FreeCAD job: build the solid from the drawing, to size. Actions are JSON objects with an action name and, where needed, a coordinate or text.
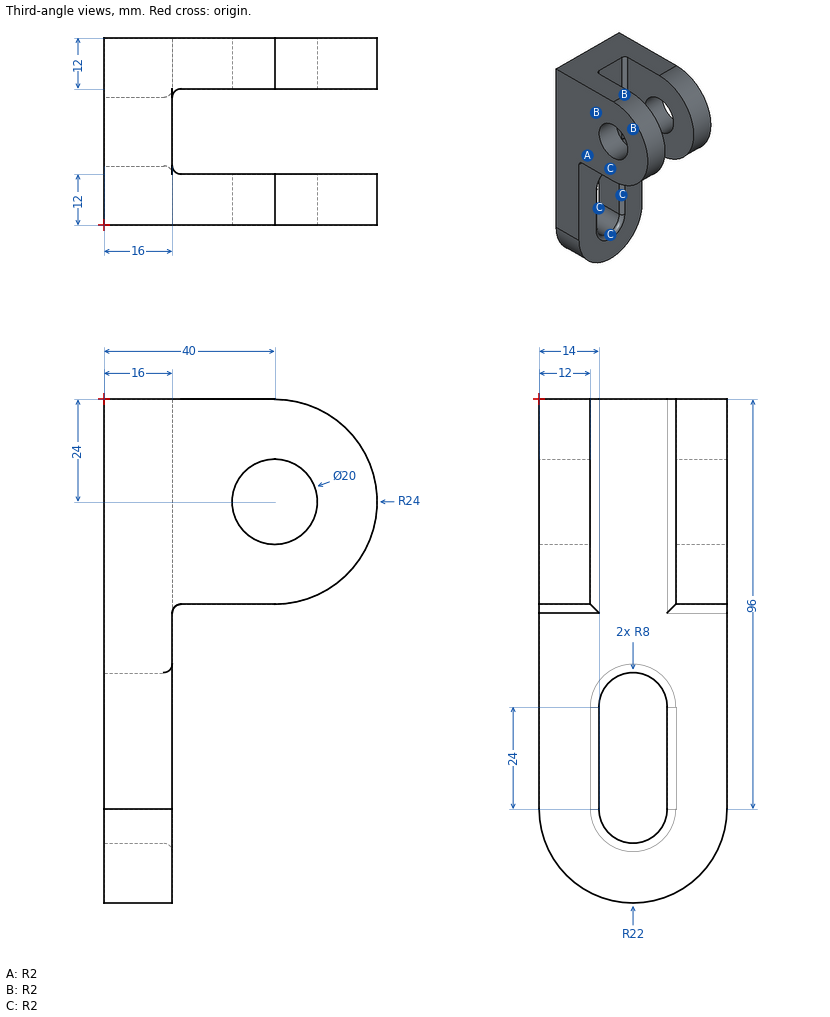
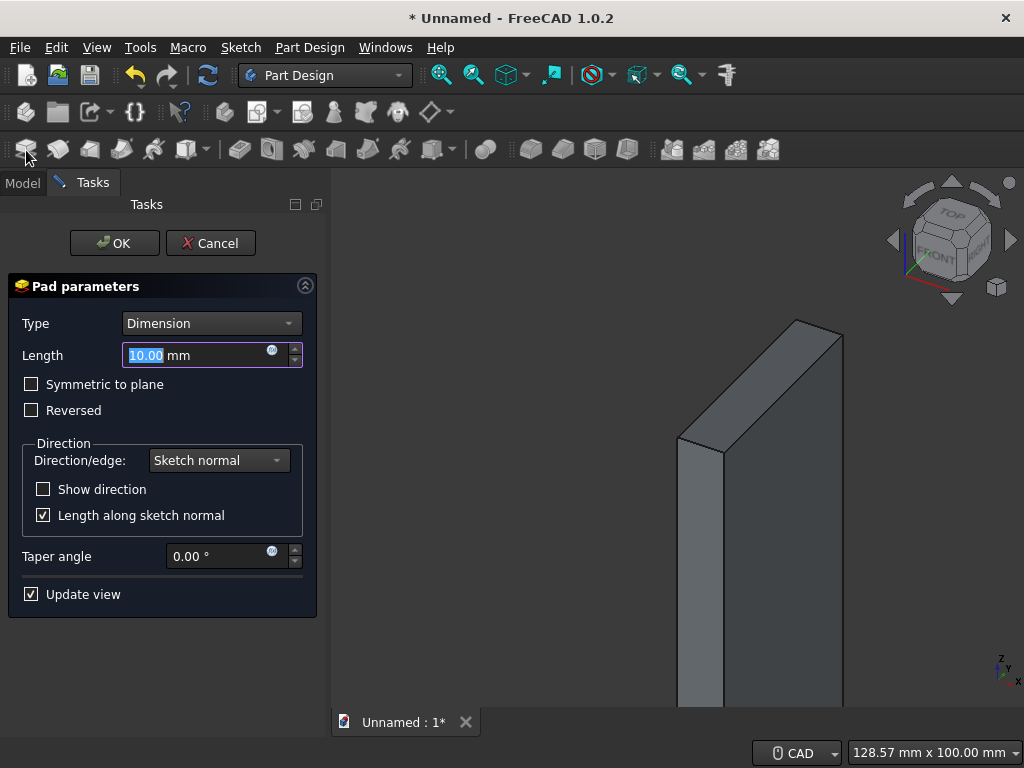
{"action": "type", "text": "16"}
{"action": "key", "text": "Tab"}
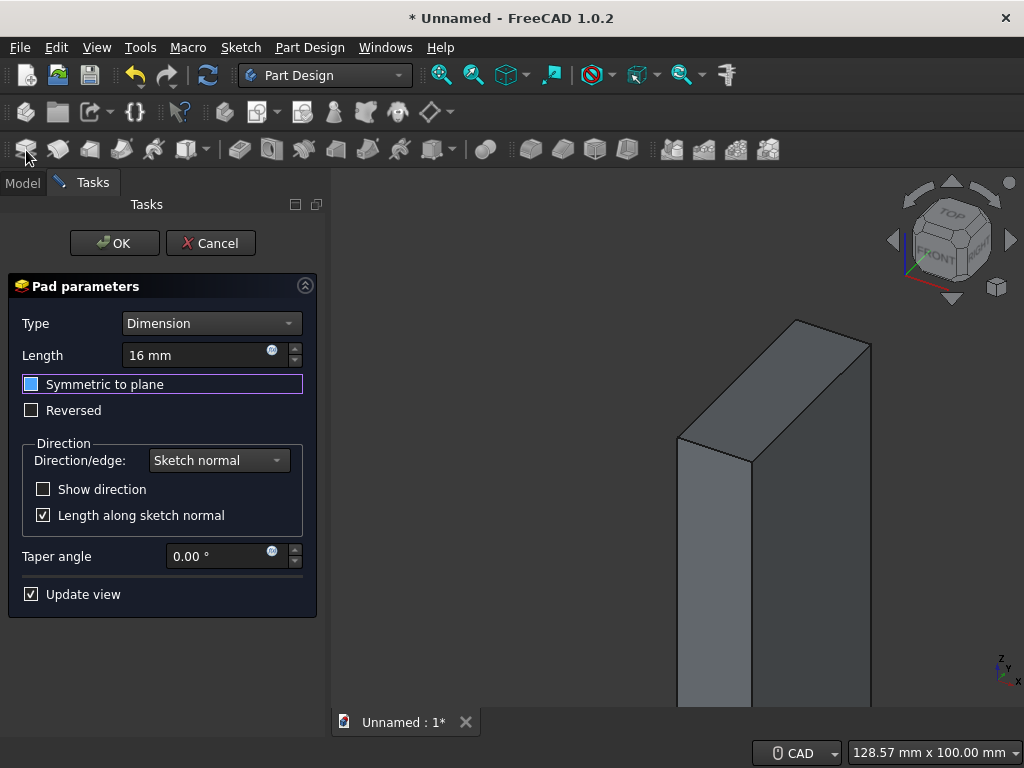
{"action": "left_click", "coordinate": [115, 243]}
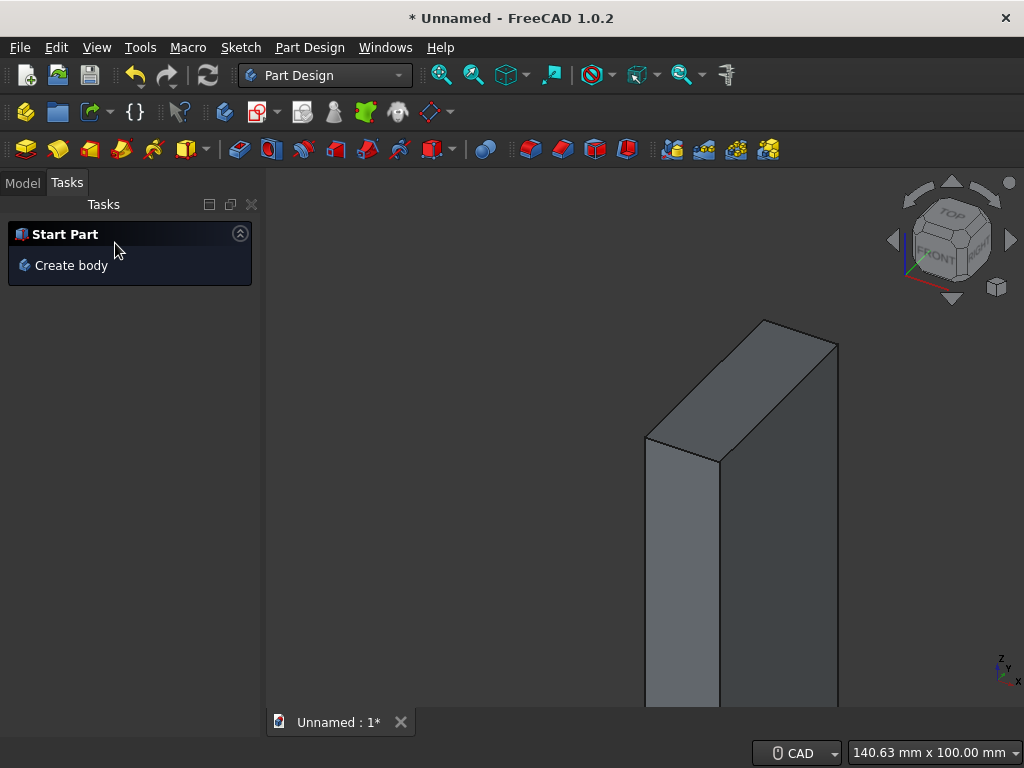
{"action": "left_click", "coordinate": [442, 76]}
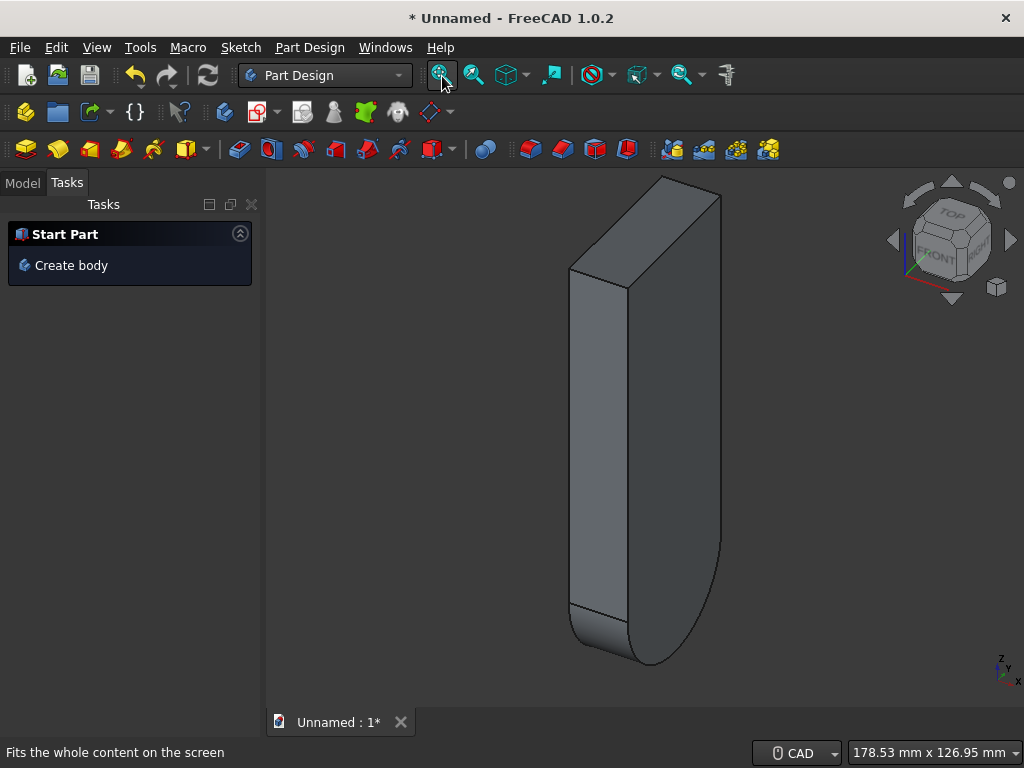
{"action": "left_click", "coordinate": [674, 563]}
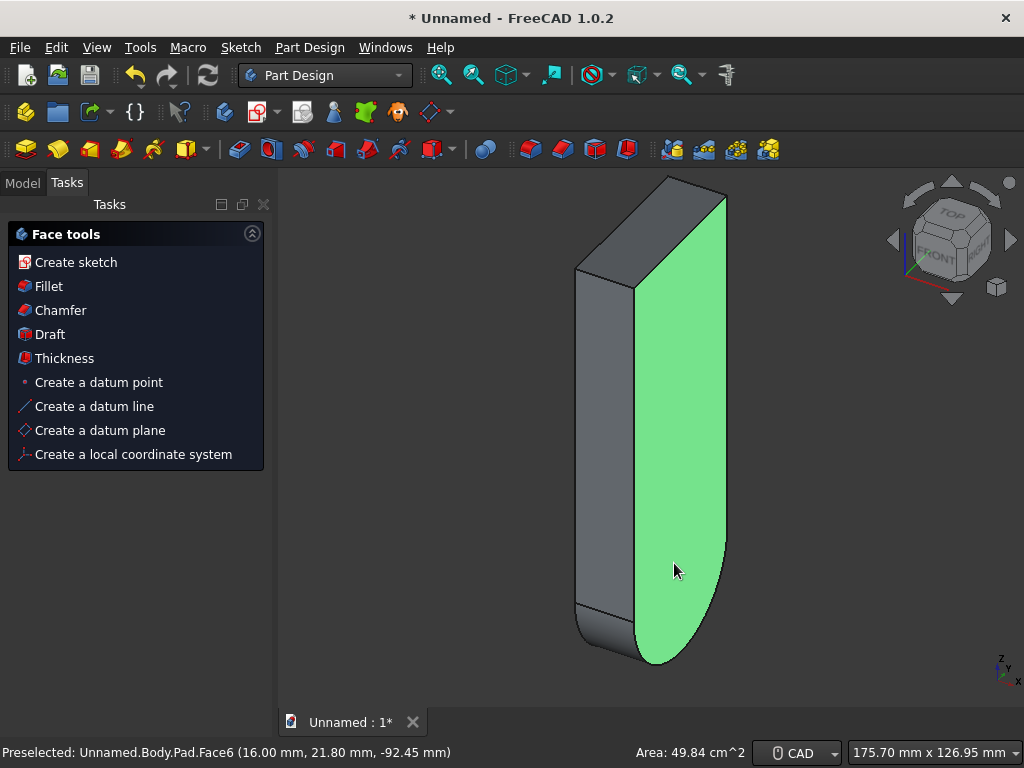
{"action": "left_click", "coordinate": [258, 112]}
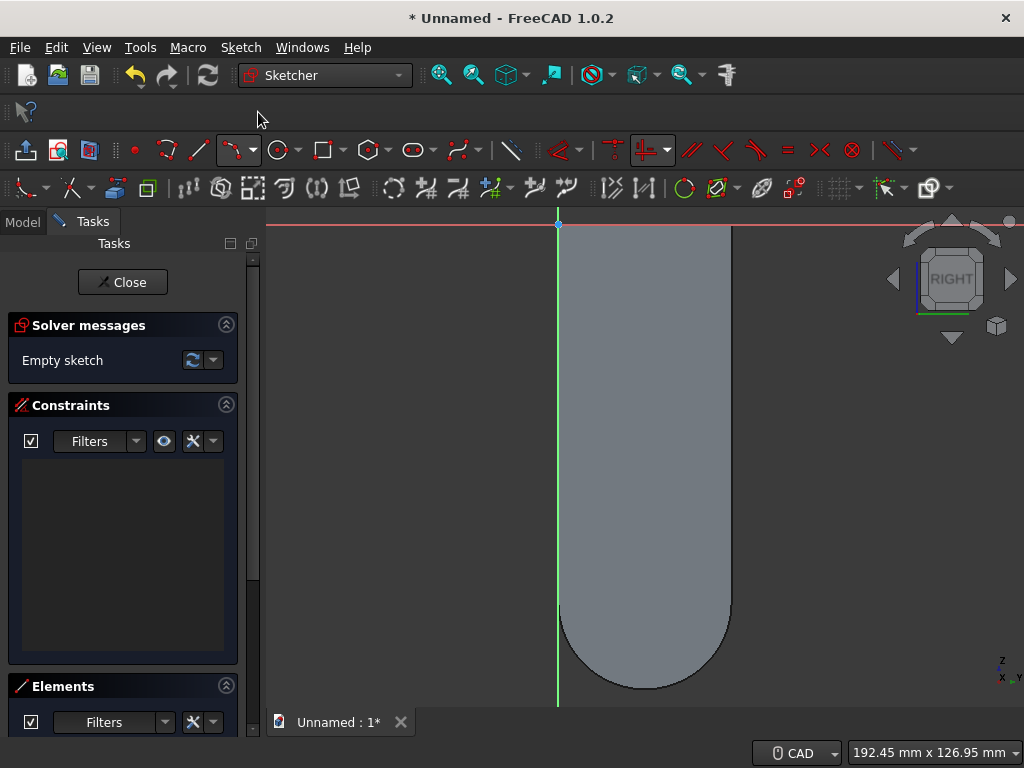
{"action": "scroll", "coordinate": [728, 675], "scroll_direction": "up", "scroll_amount": 3}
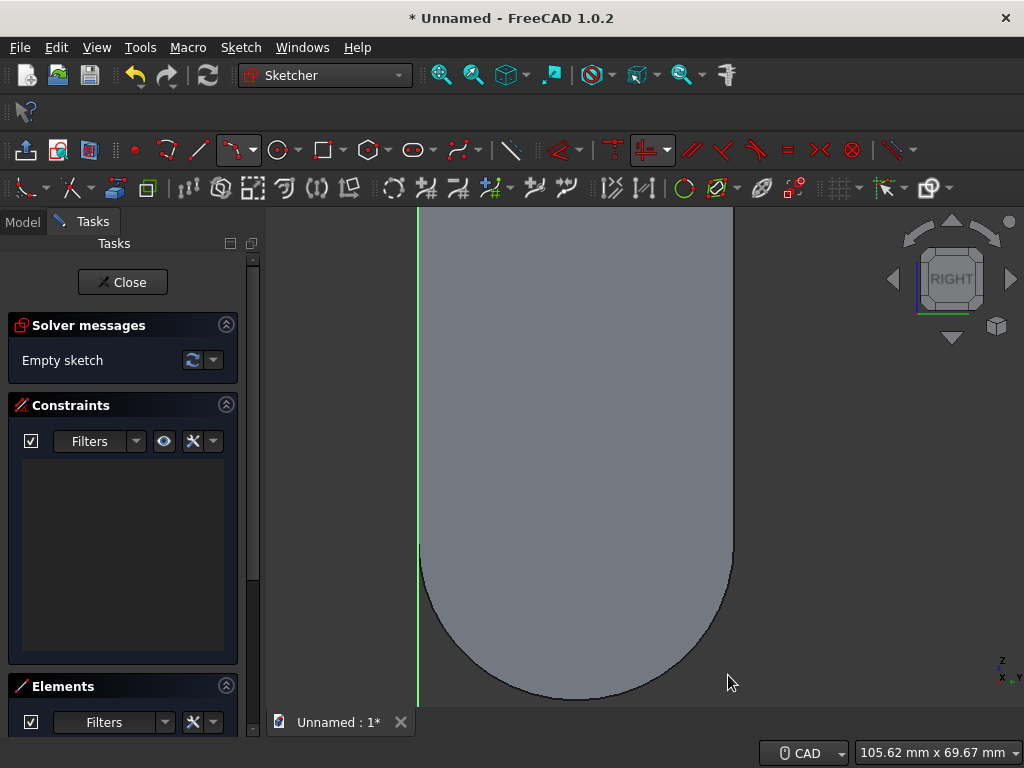
{"action": "left_click", "coordinate": [414, 150]}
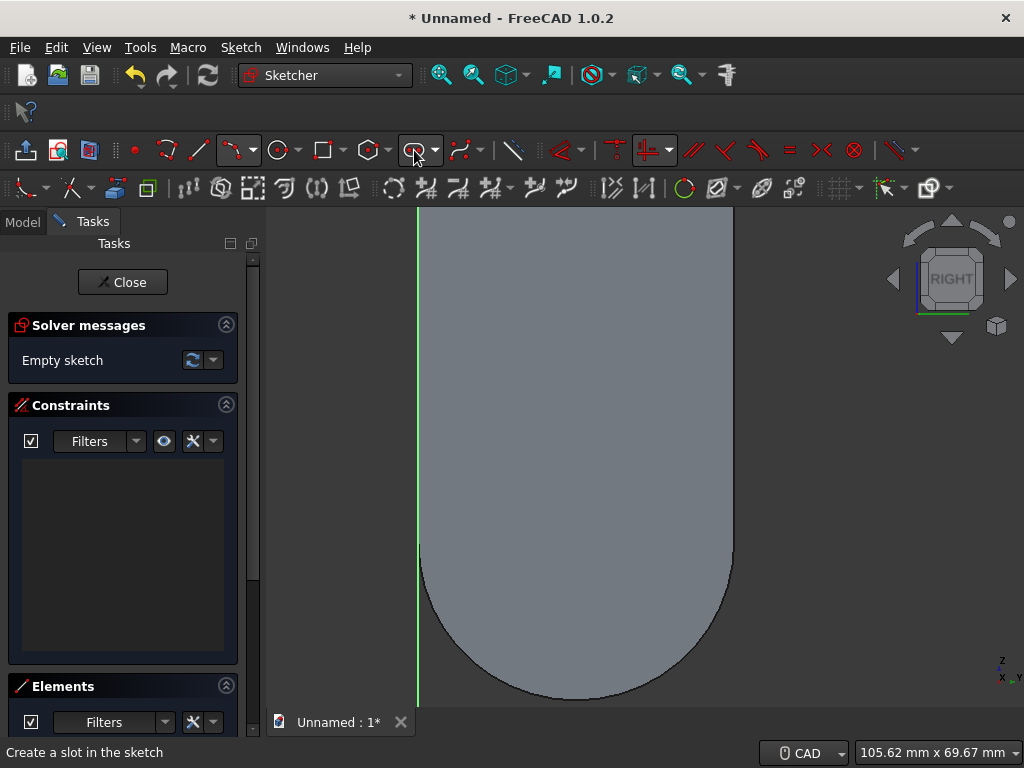
{"action": "left_click", "coordinate": [576, 543]}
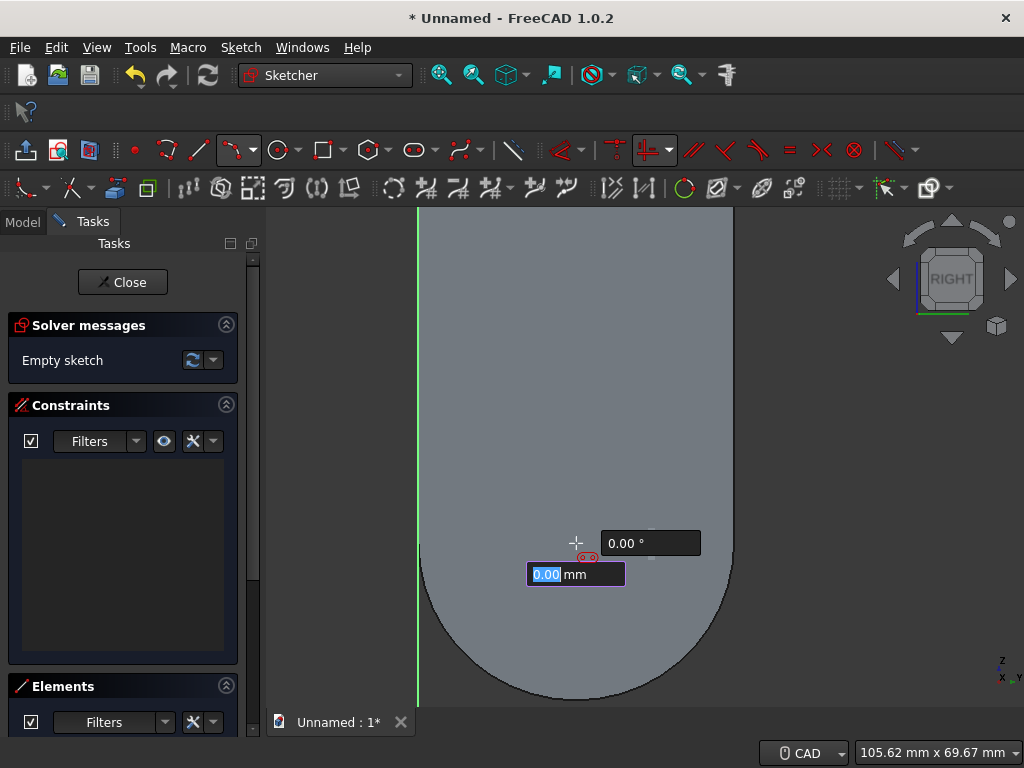
{"action": "left_click", "coordinate": [576, 370]}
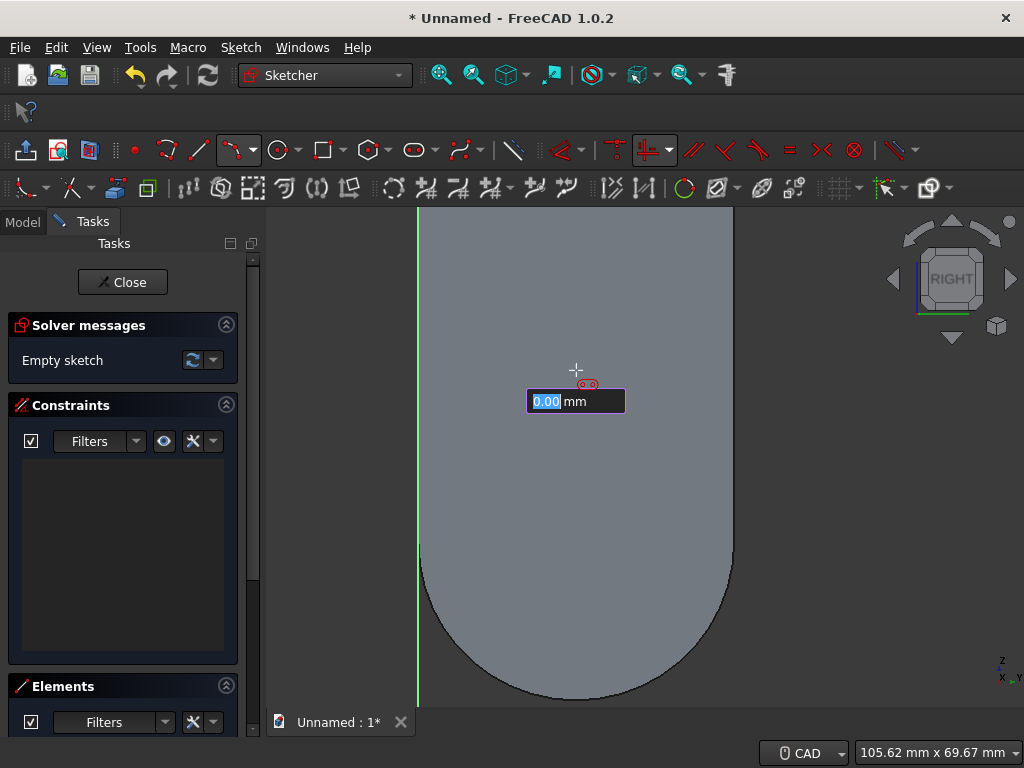
{"action": "left_click", "coordinate": [634, 456]}
{"action": "key", "text": "Escape"}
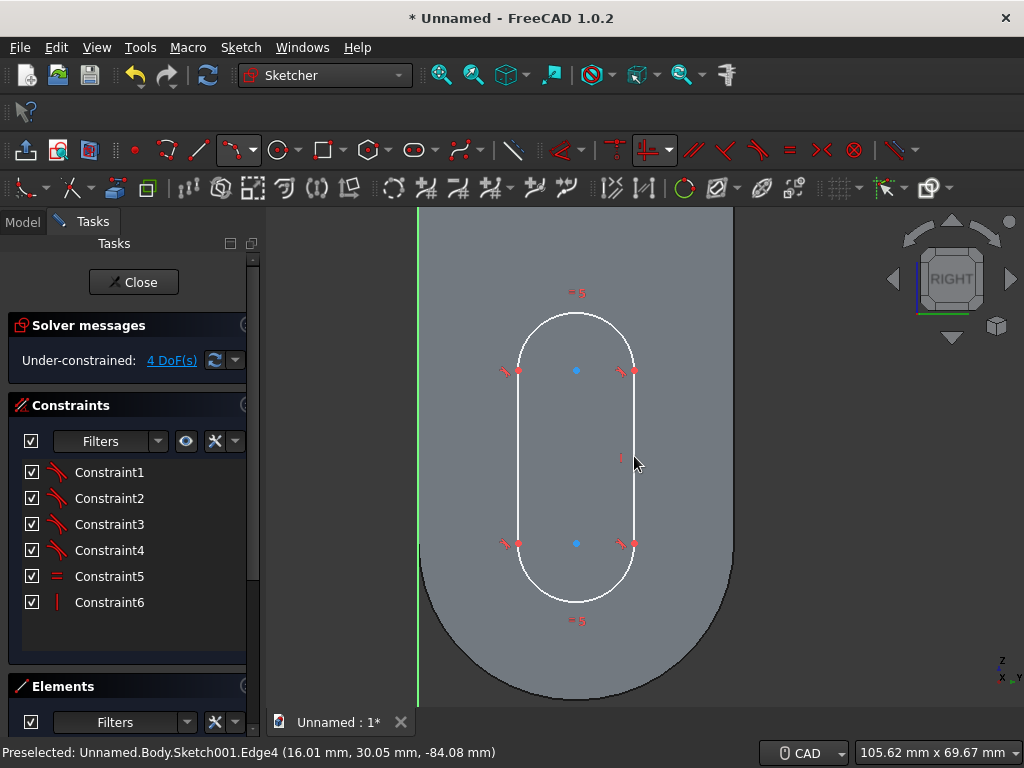
{"action": "left_click", "coordinate": [560, 150]}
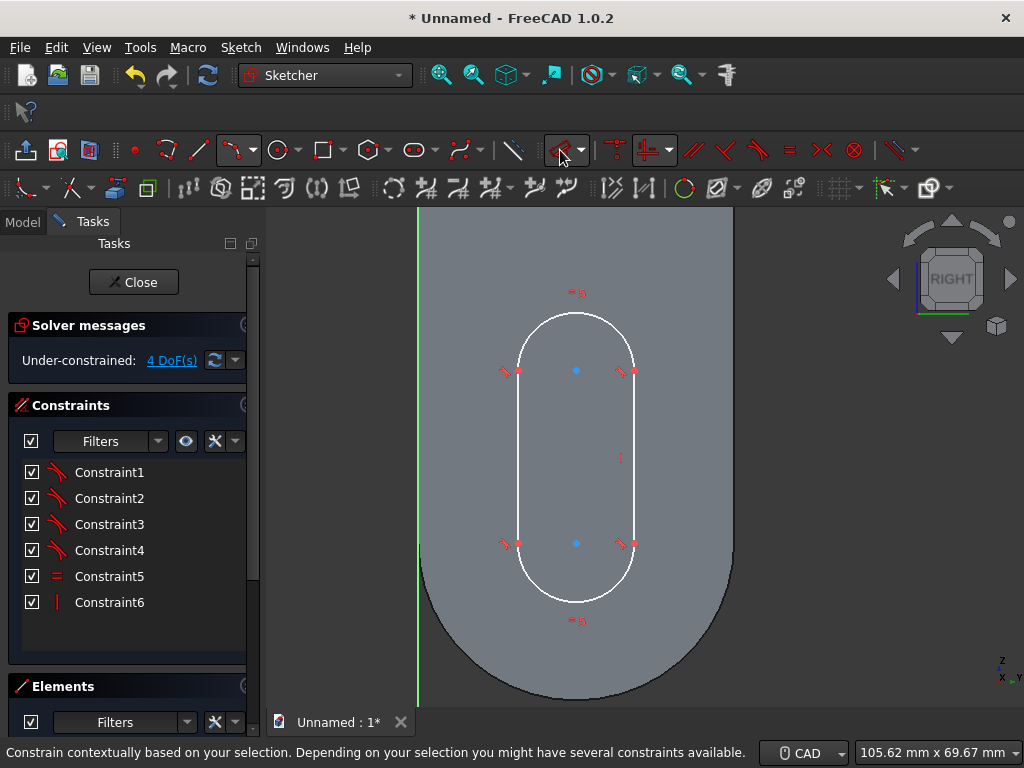
{"action": "left_click", "coordinate": [542, 591]}
{"action": "left_click", "coordinate": [523, 617]}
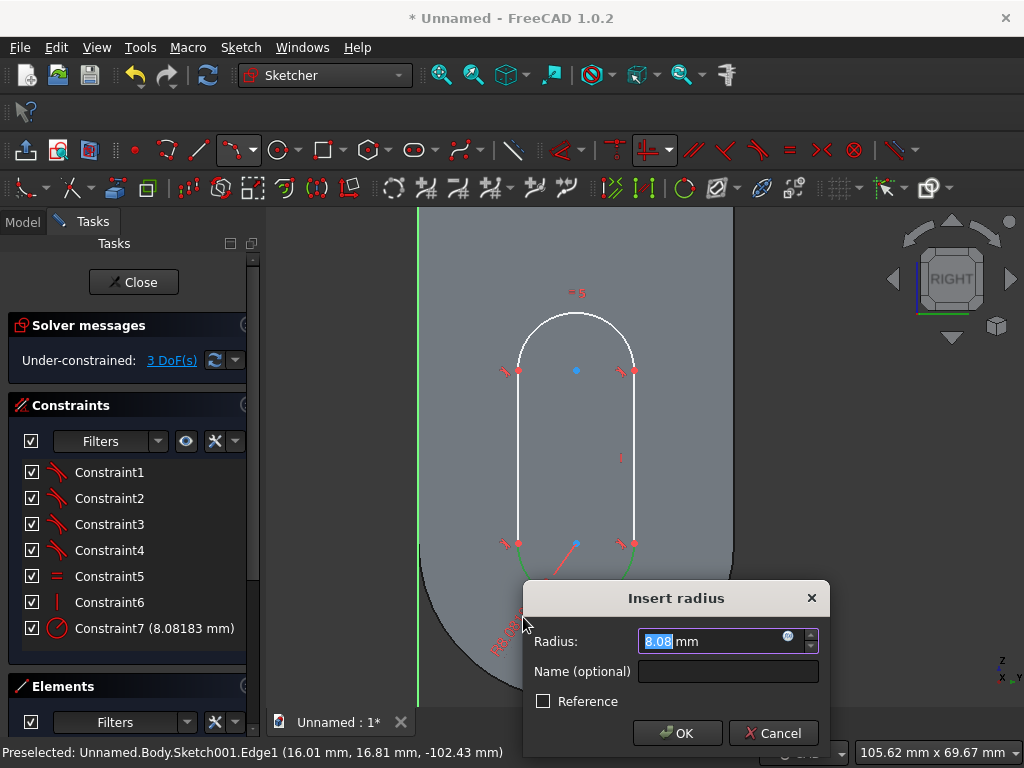
{"action": "type", "text": "8"}
{"action": "key", "text": "Return"}